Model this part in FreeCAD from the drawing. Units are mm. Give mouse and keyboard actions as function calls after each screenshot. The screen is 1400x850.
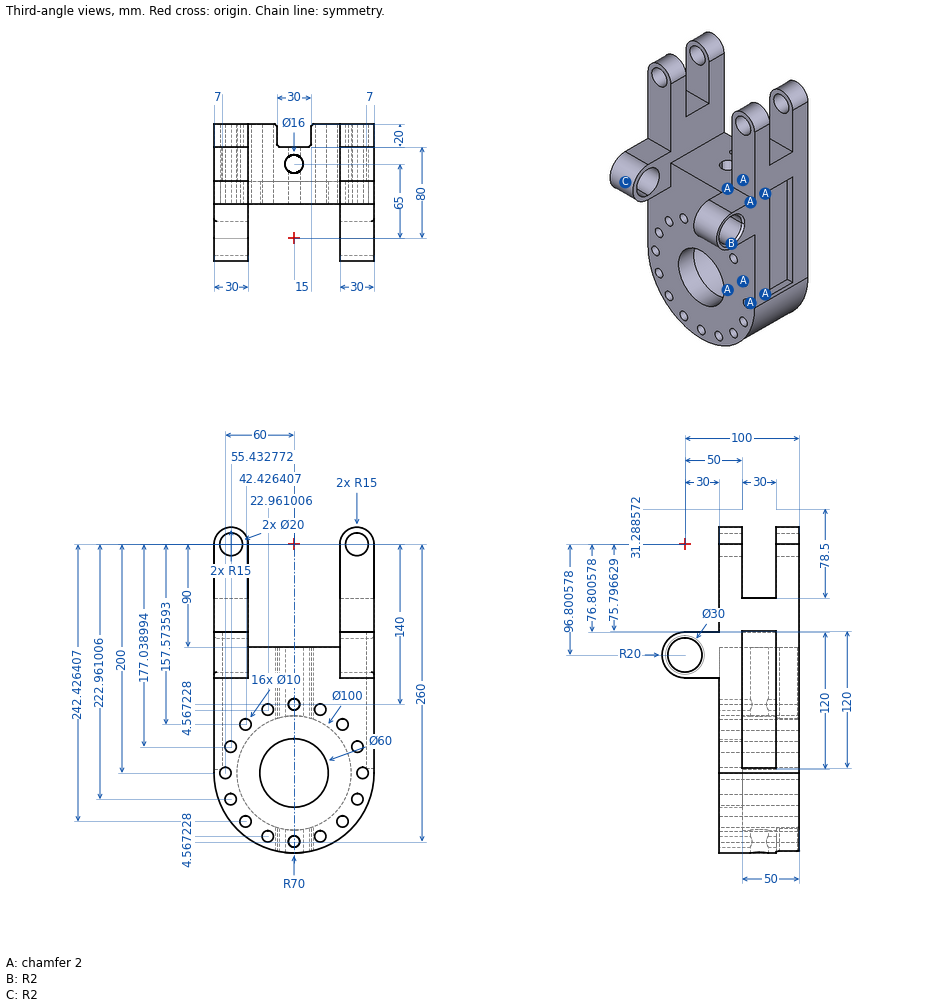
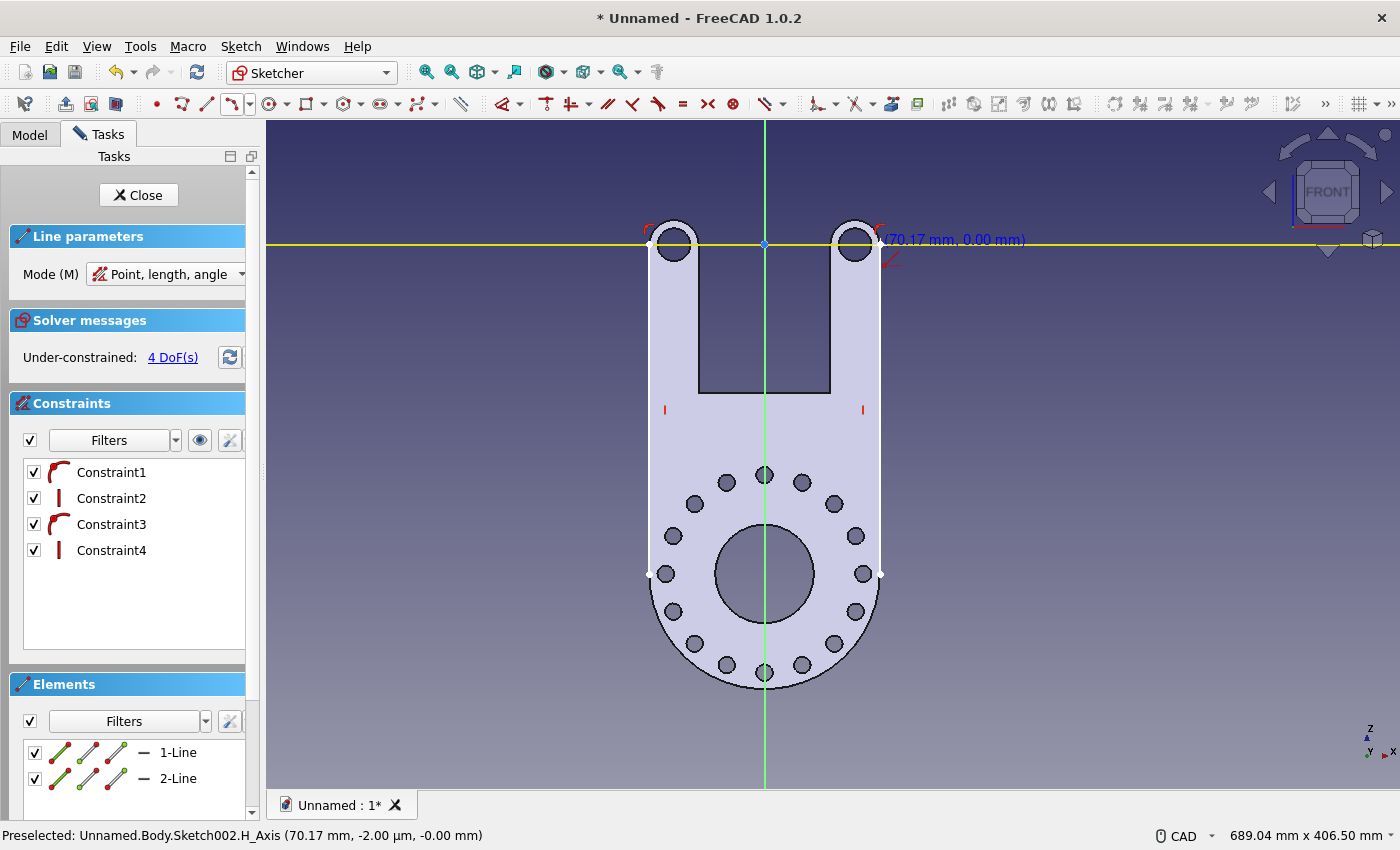
key(g)
key(m)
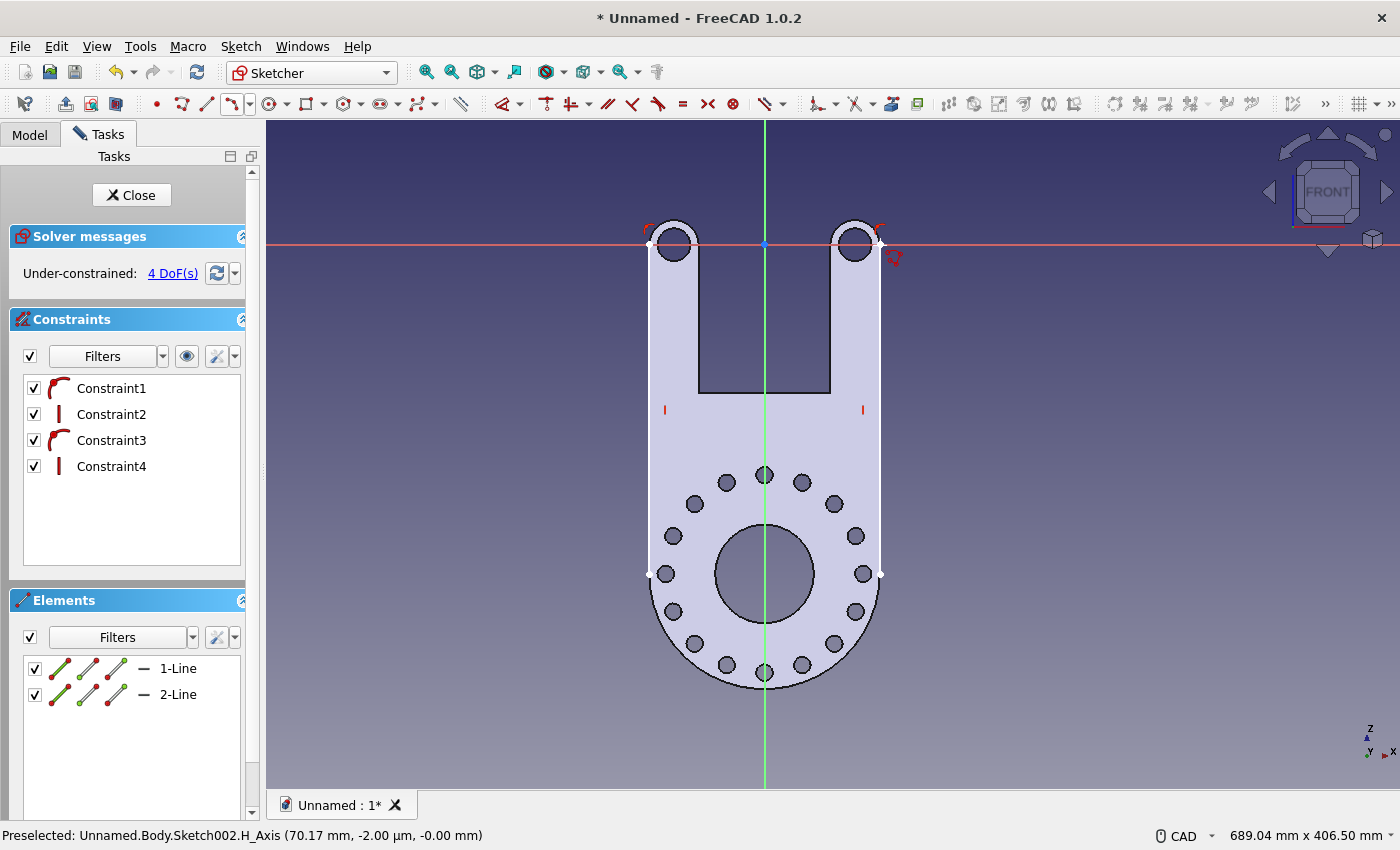
click(830, 245)
click(830, 393)
click(699, 393)
click(699, 245)
right_click(699, 245)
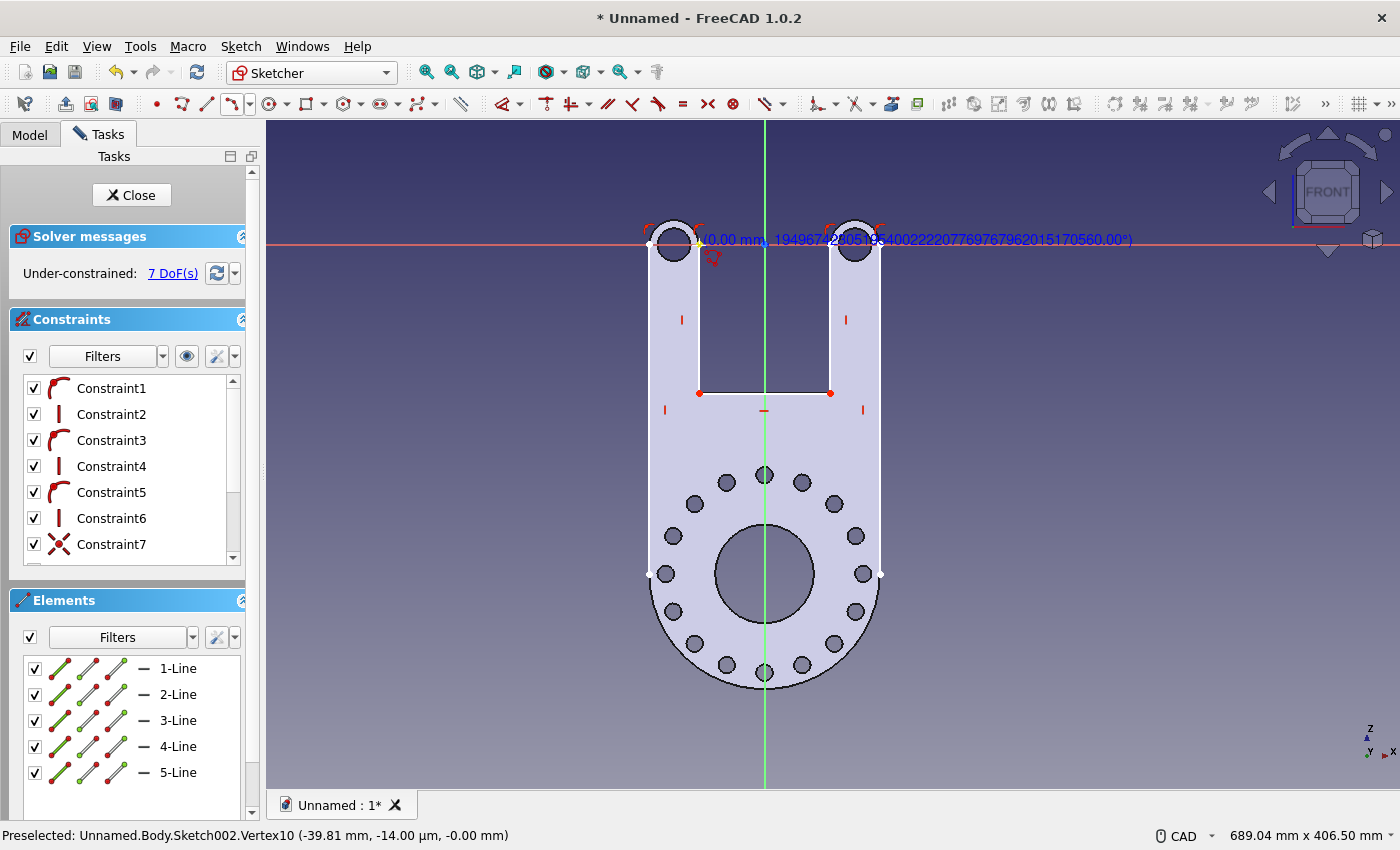
key(g)
key(3)
key(a)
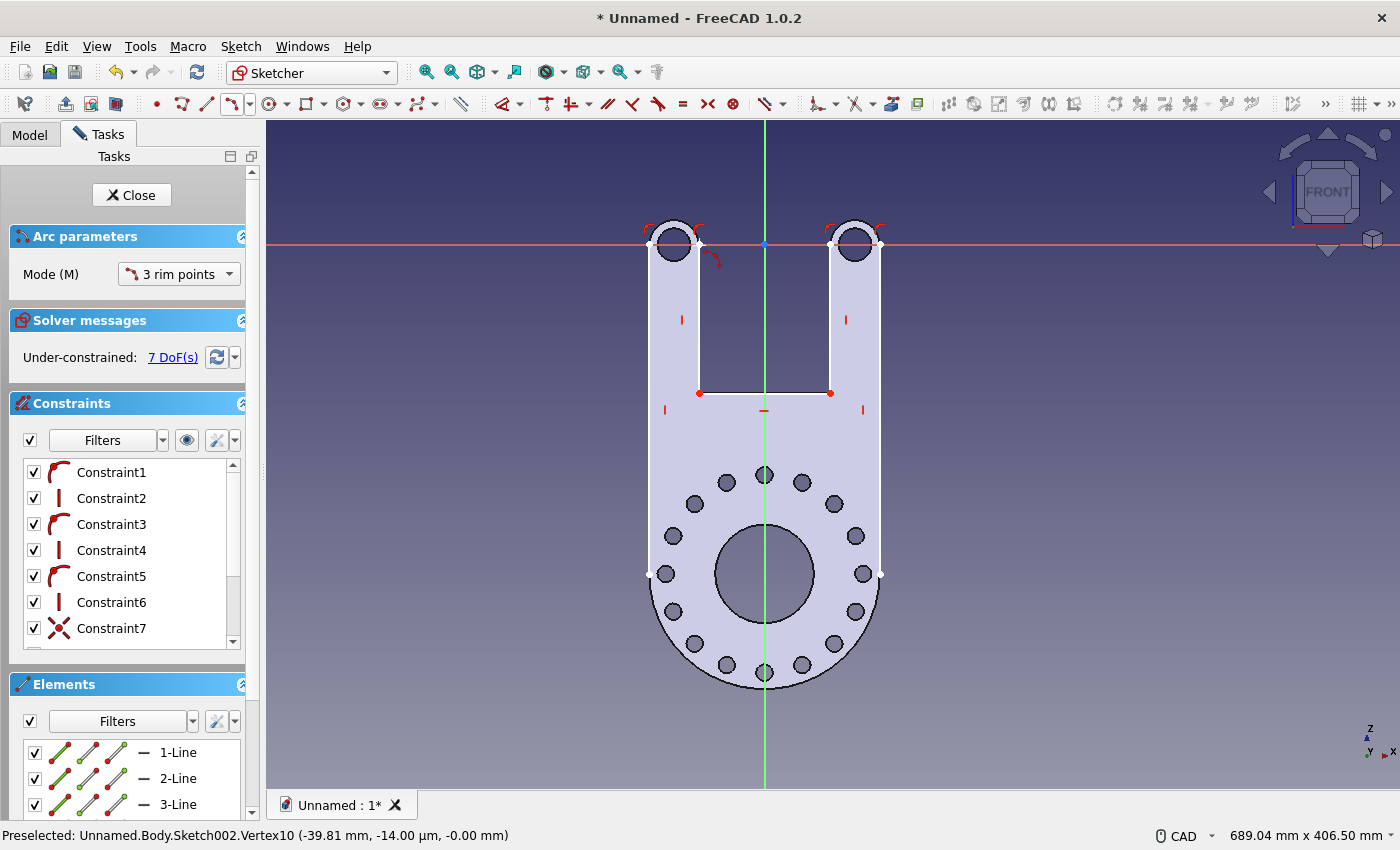
click(649, 575)
click(880, 575)
click(729, 683)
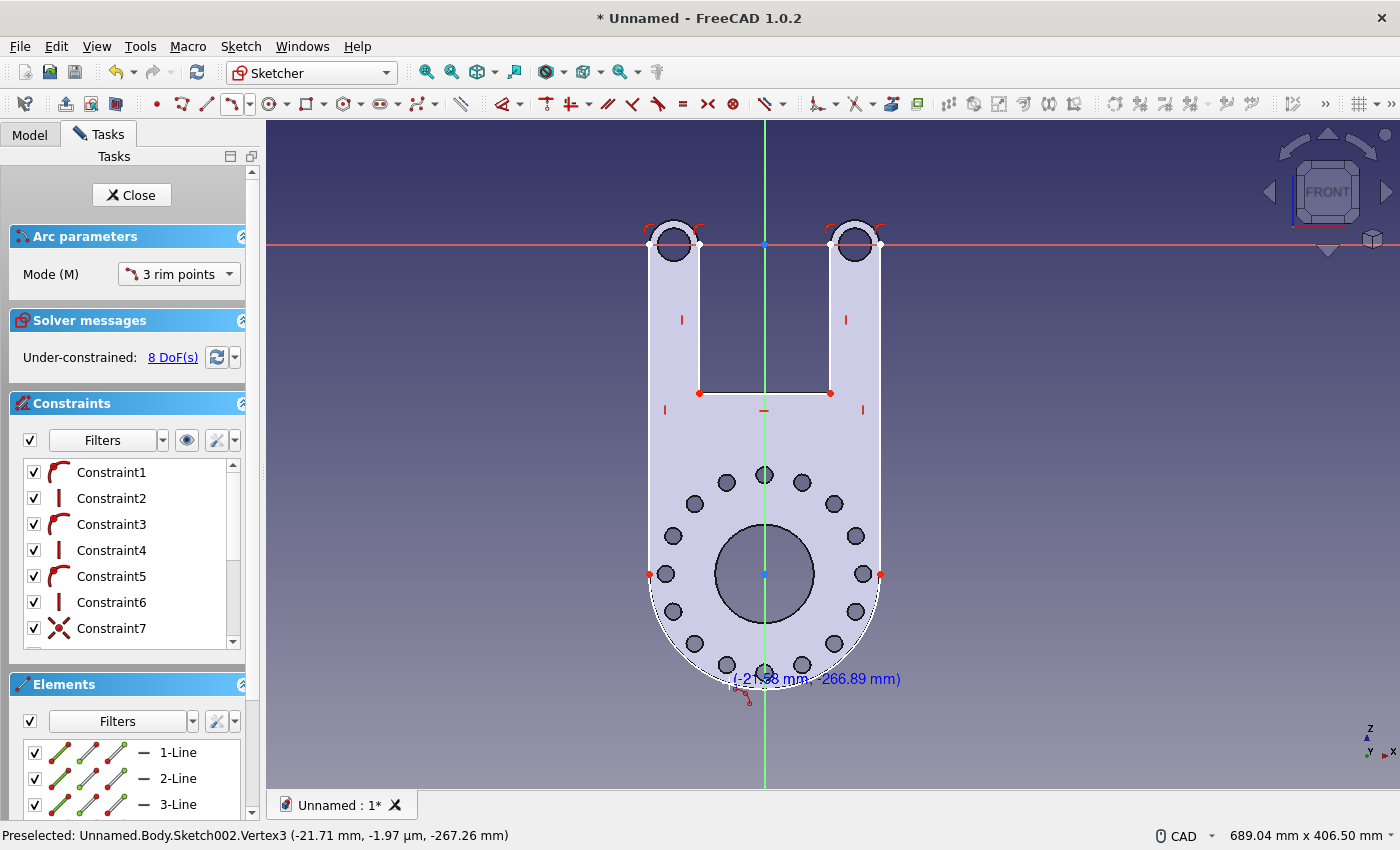
click(880, 245)
click(830, 245)
click(855, 220)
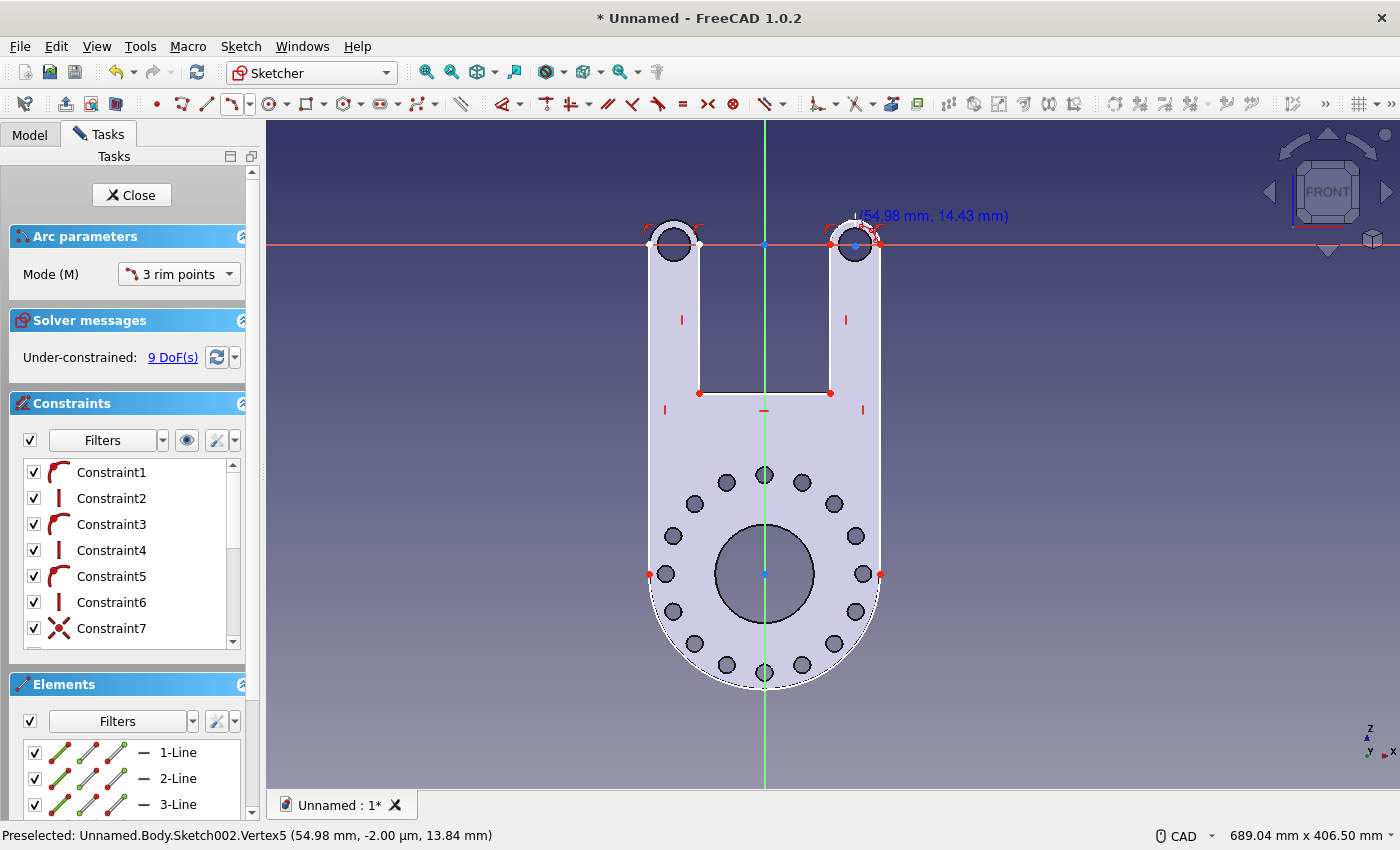
click(699, 245)
click(649, 245)
click(674, 220)
key(Escape)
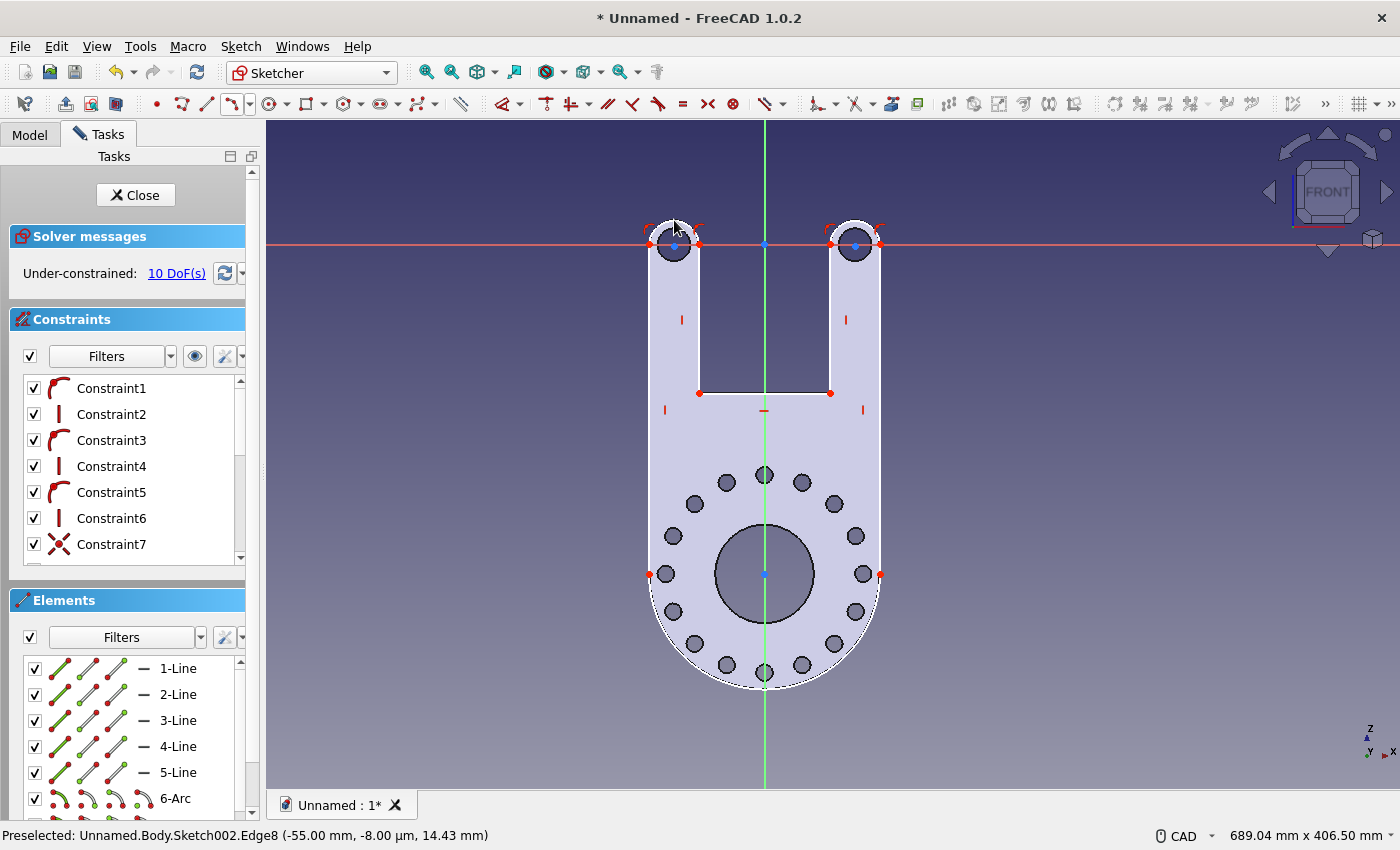
click(649, 344)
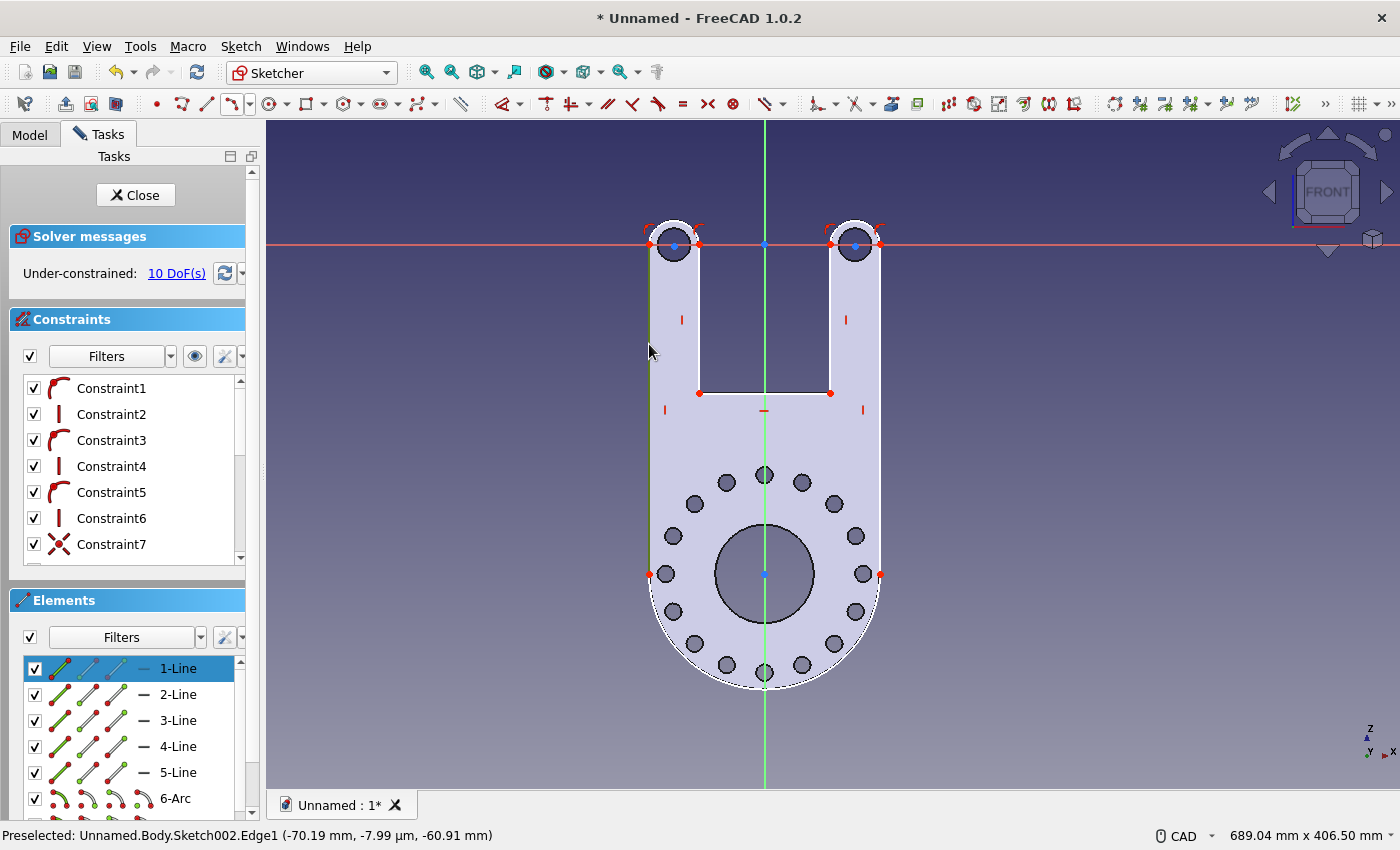
click(688, 225)